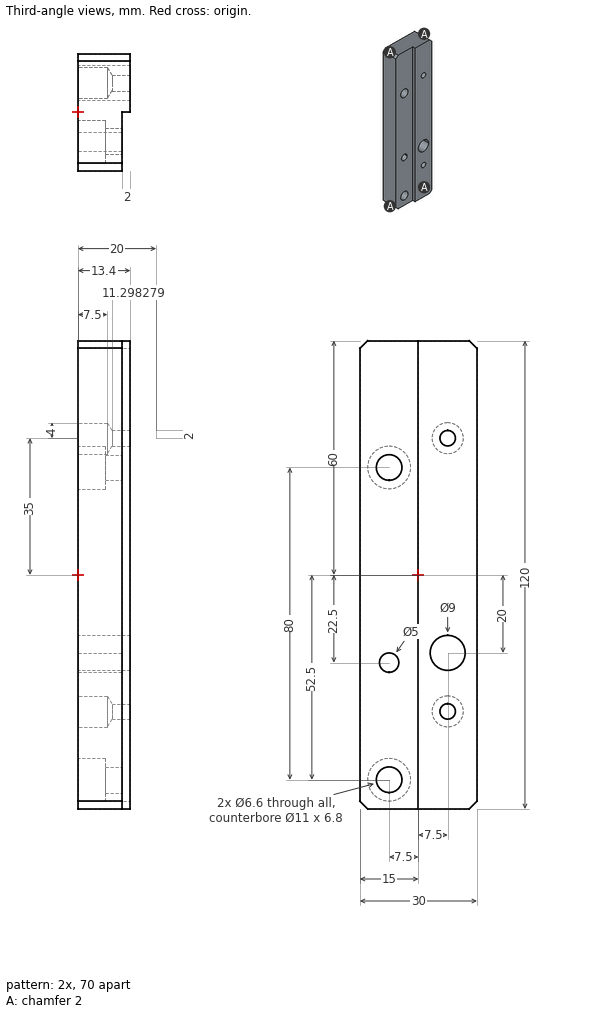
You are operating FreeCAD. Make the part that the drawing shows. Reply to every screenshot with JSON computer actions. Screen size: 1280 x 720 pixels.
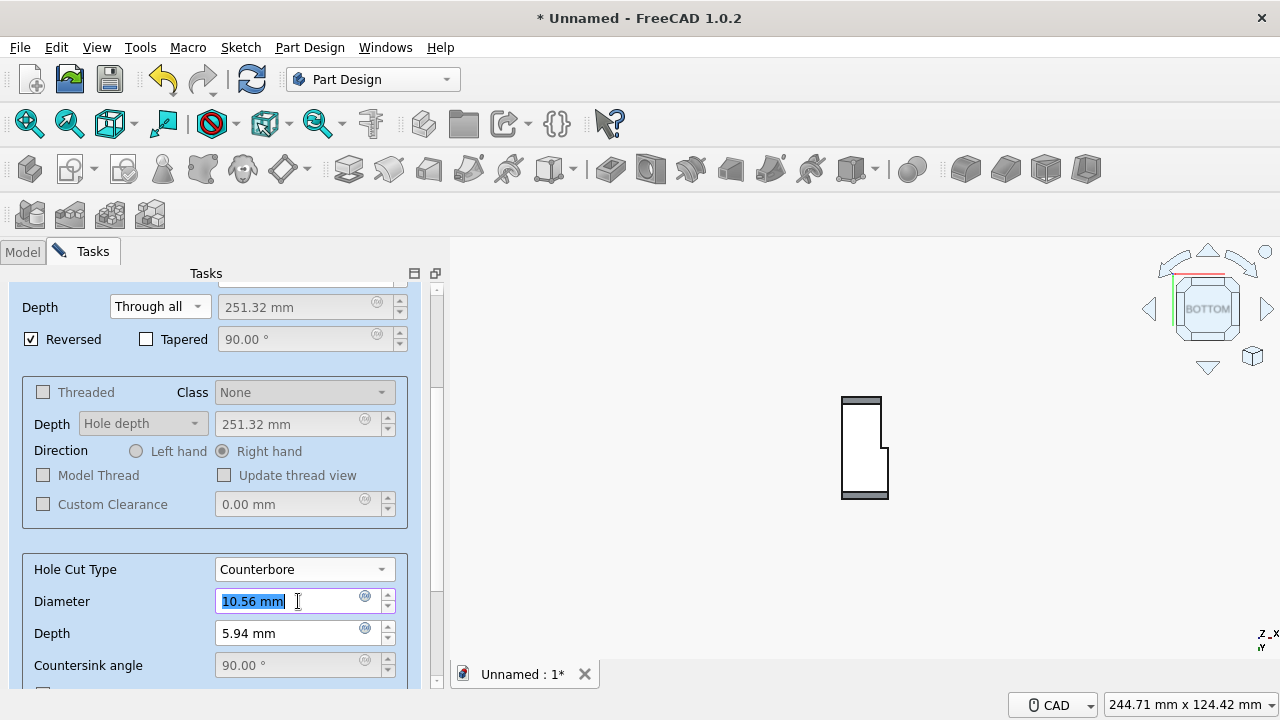
{"action": "type", "text": "11"}
{"action": "key", "text": "Tab"}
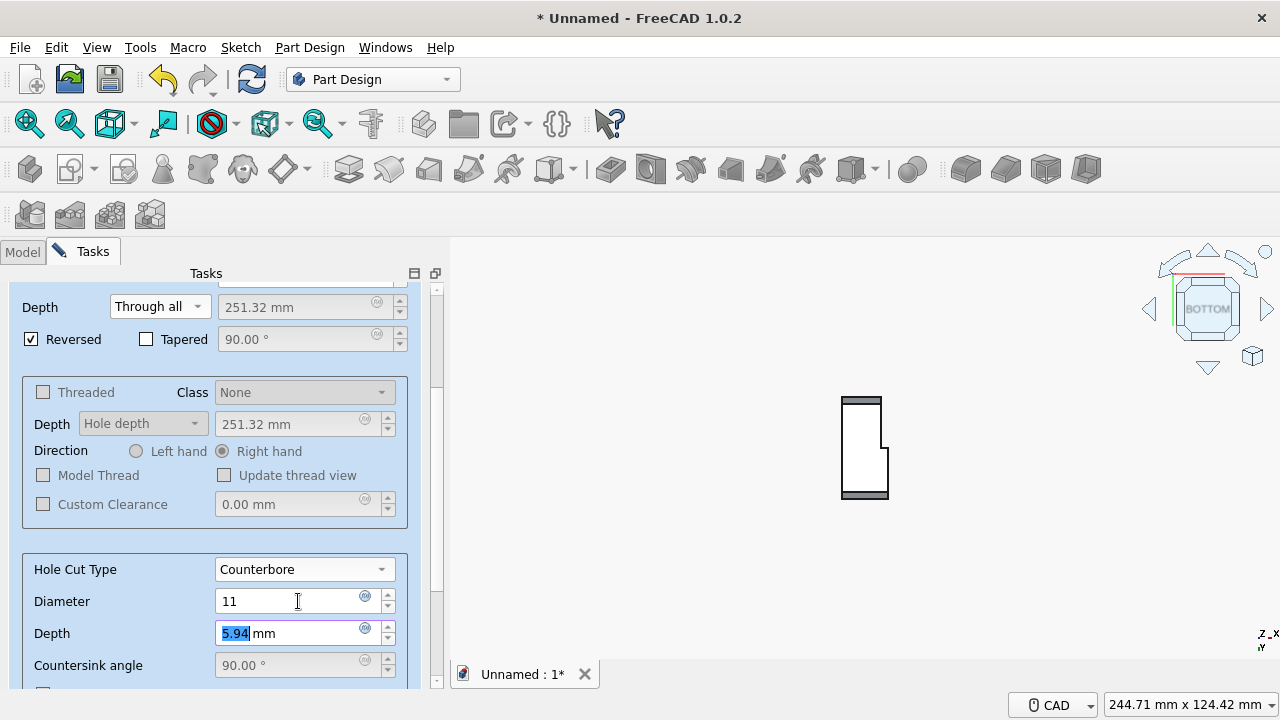
{"action": "type", "text": "6.8"}
{"action": "key", "text": "Tab"}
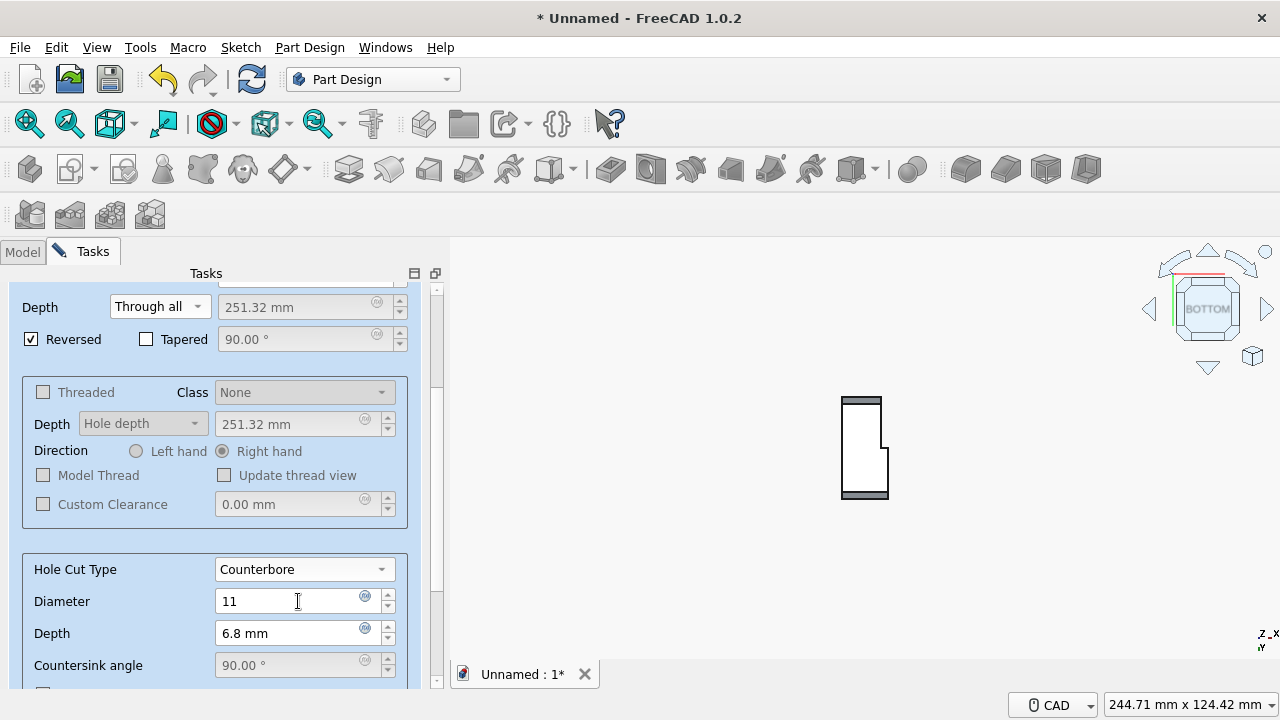
{"action": "scroll", "coordinate": [437, 486], "scroll_direction": "up", "scroll_amount": 4}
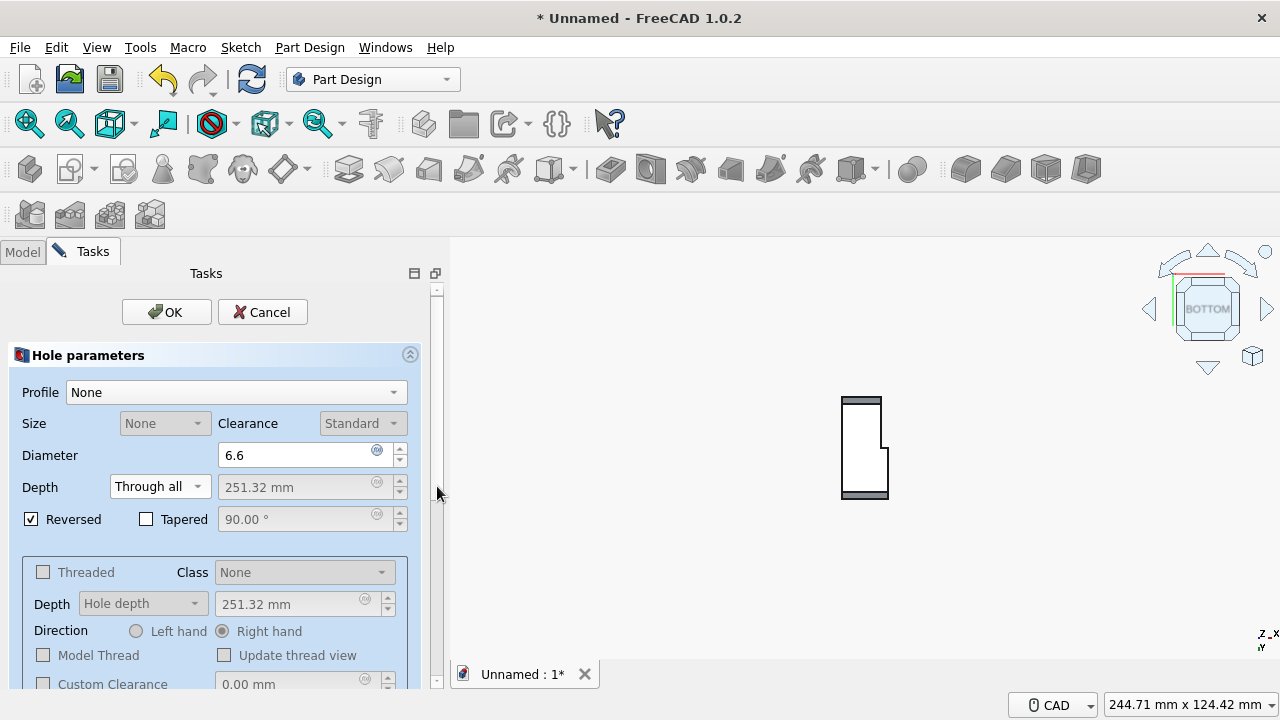
{"action": "left_click", "coordinate": [167, 312]}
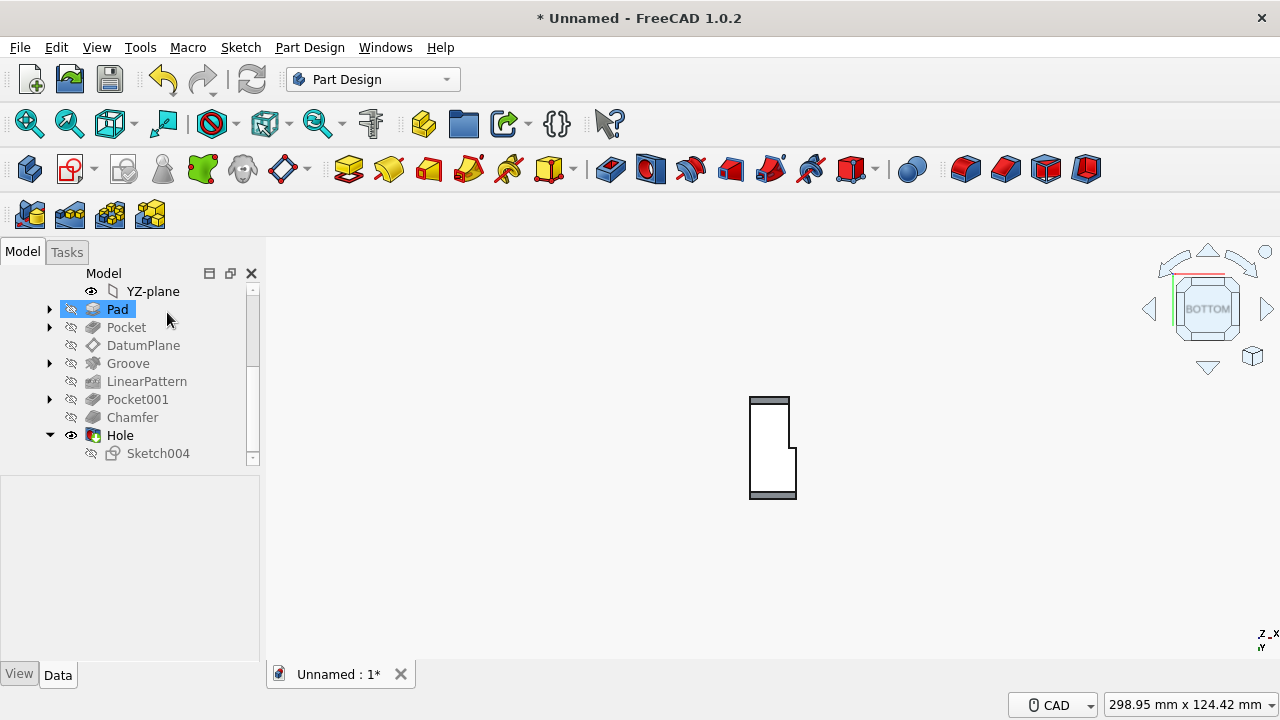
{"action": "left_click", "coordinate": [30, 124]}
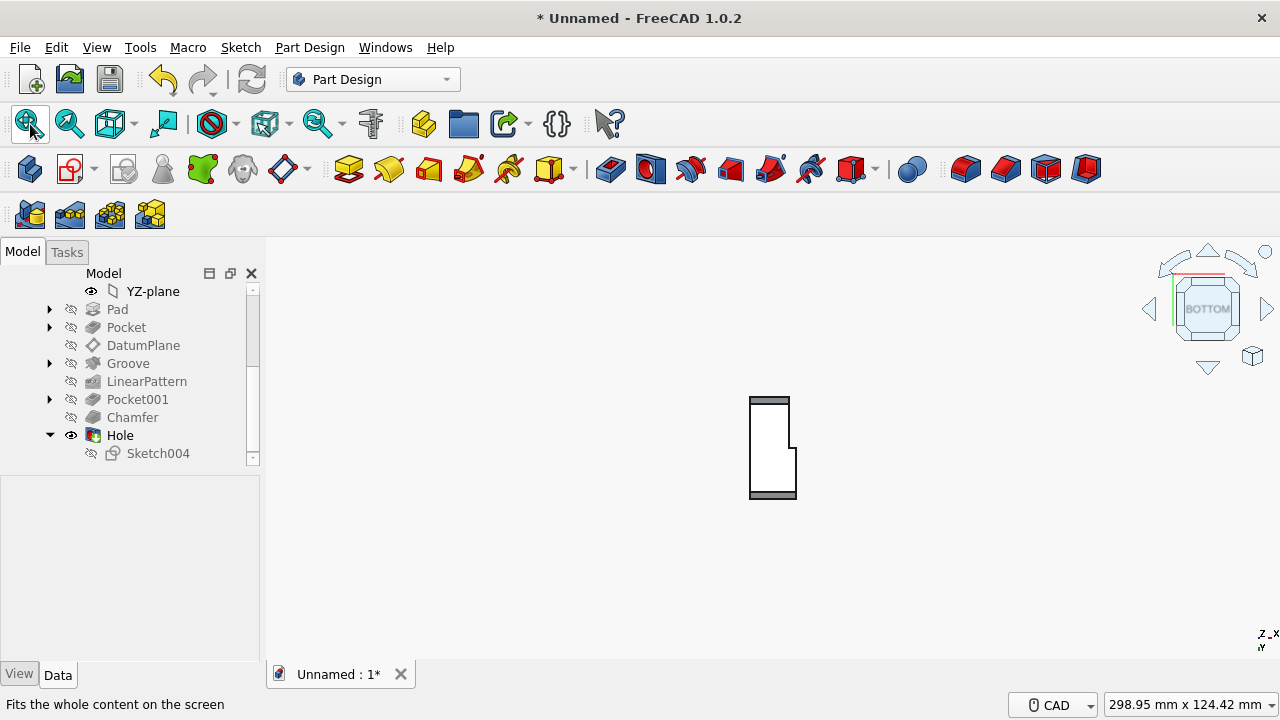
{"action": "key", "text": "6"}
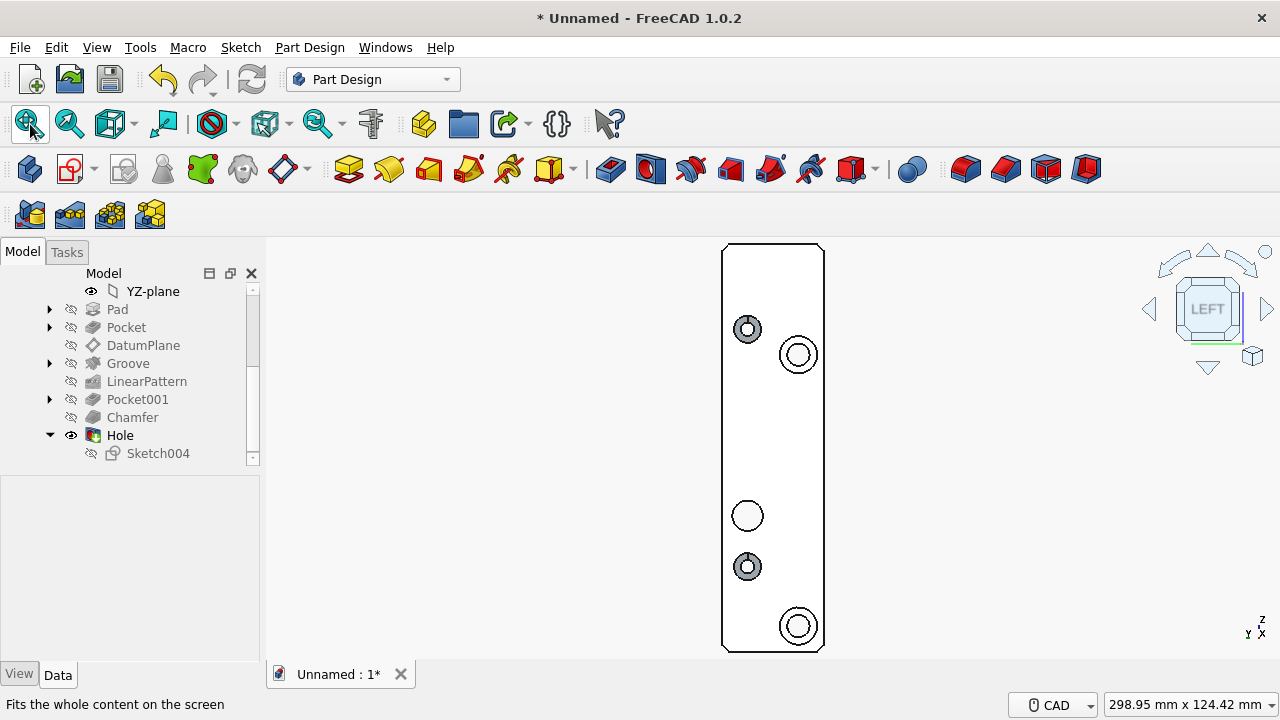
{"action": "left_click", "coordinate": [773, 447]}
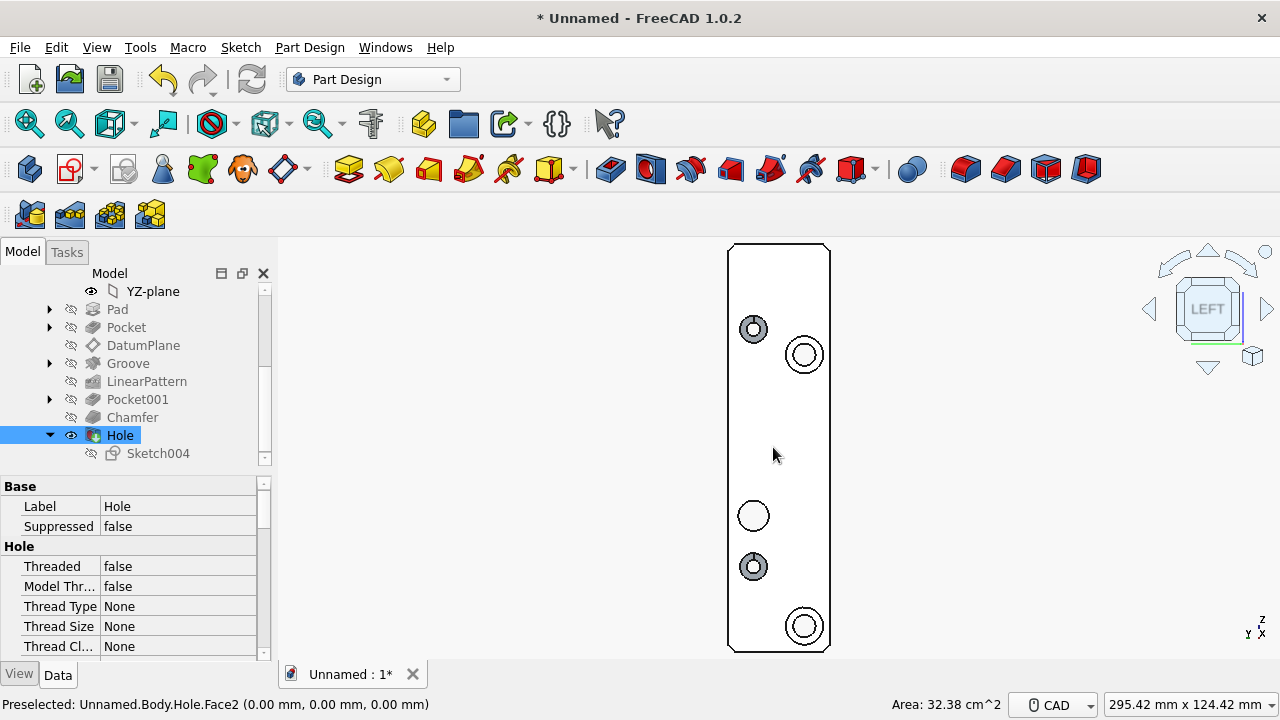
{"action": "left_click", "coordinate": [70, 170]}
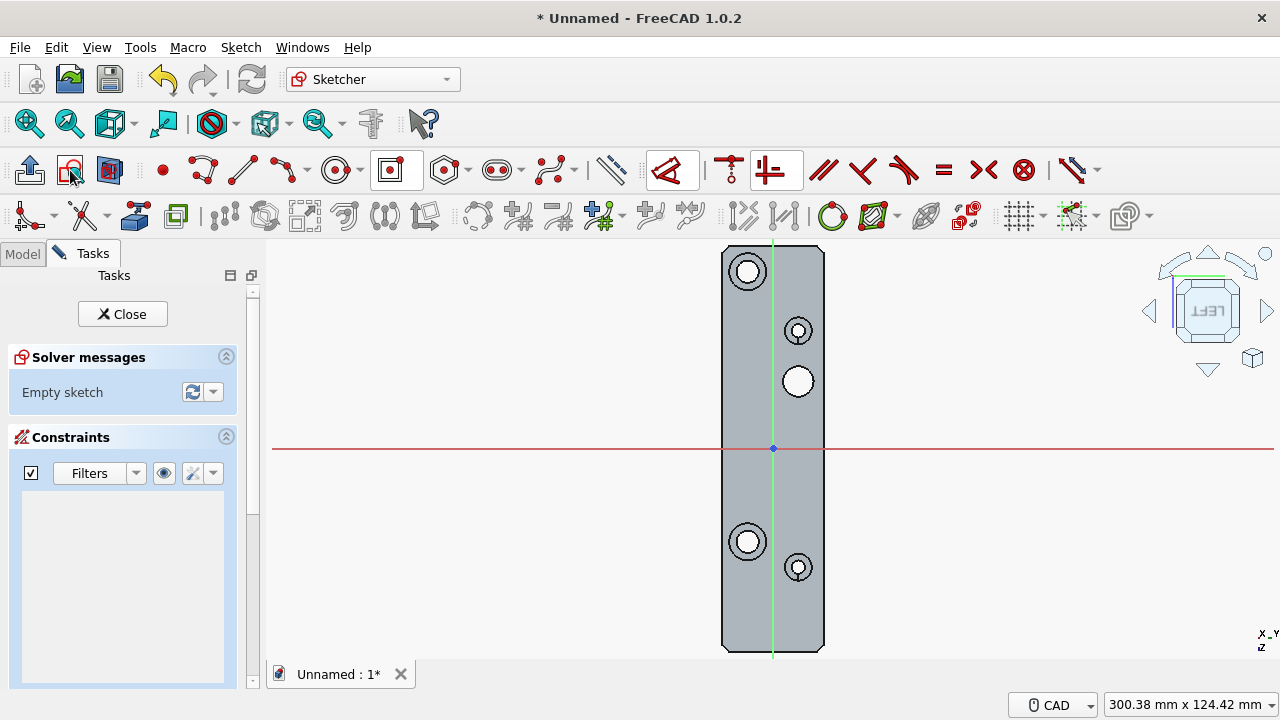
{"action": "scroll", "coordinate": [750, 368], "scroll_direction": "up", "scroll_amount": 14}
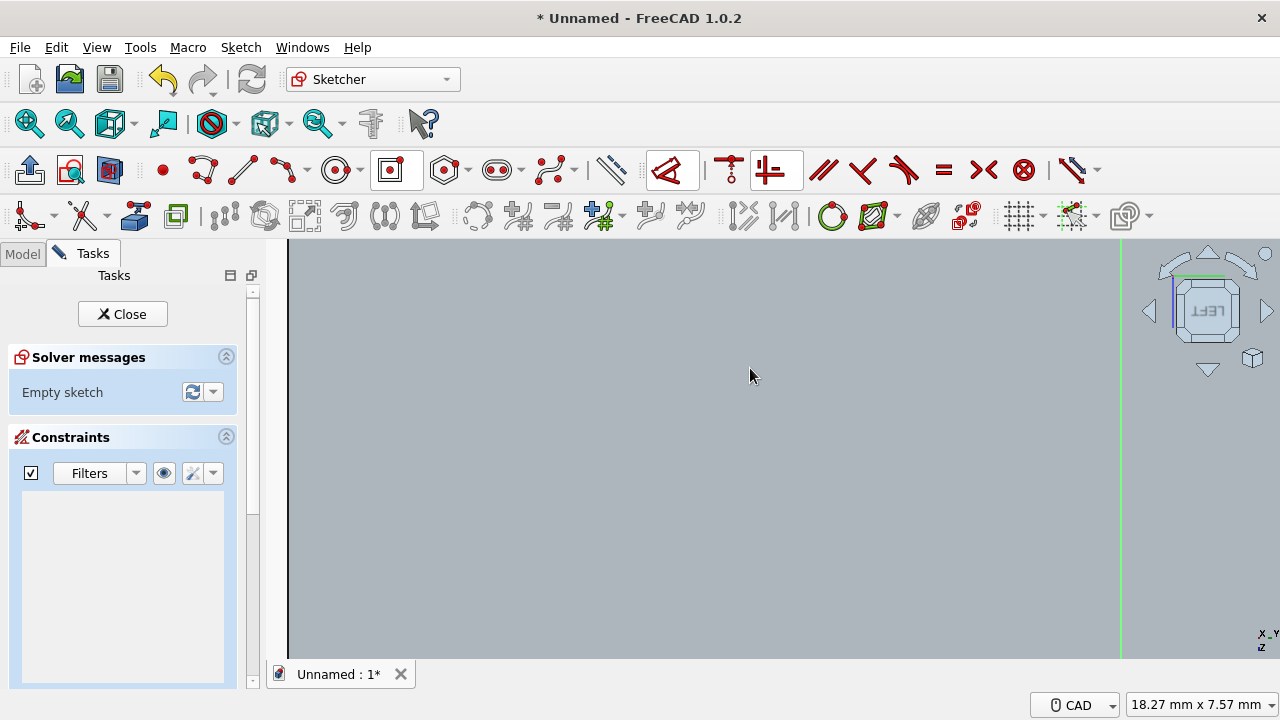
{"action": "left_click", "coordinate": [336, 170]}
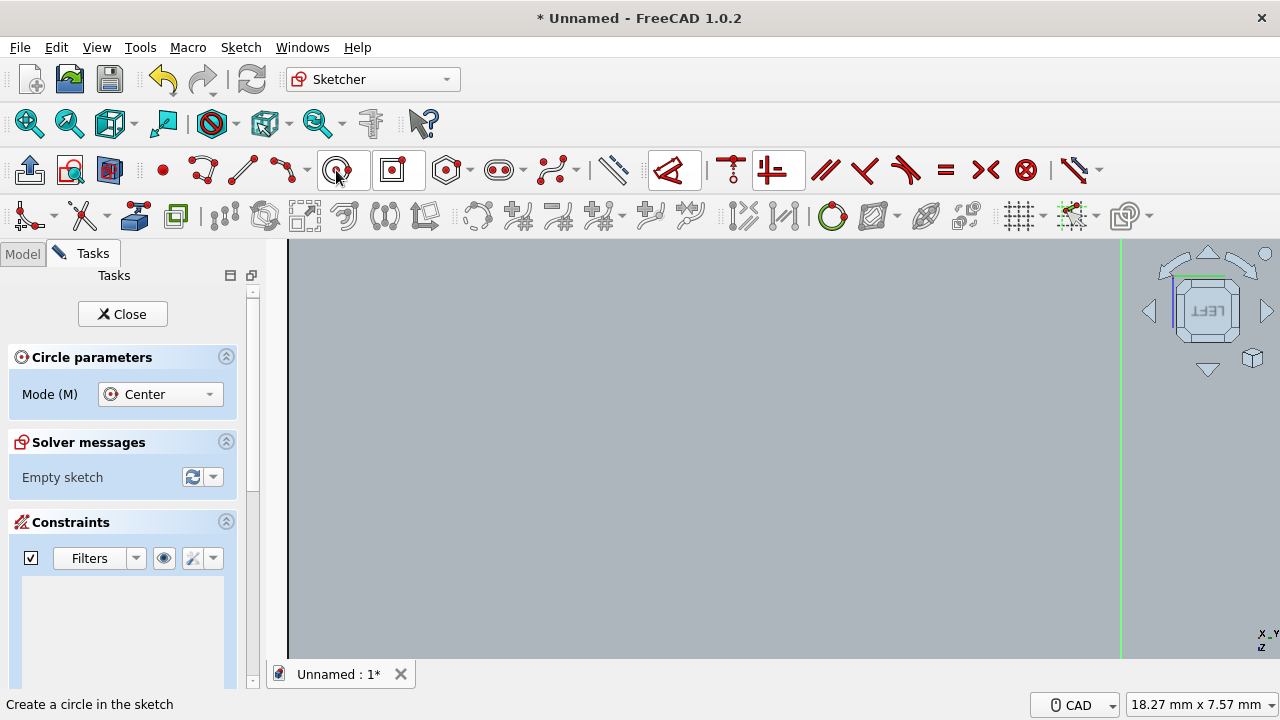
{"action": "left_click", "coordinate": [705, 446]}
{"action": "left_click", "coordinate": [803, 348]}
{"action": "key", "text": "Escape"}